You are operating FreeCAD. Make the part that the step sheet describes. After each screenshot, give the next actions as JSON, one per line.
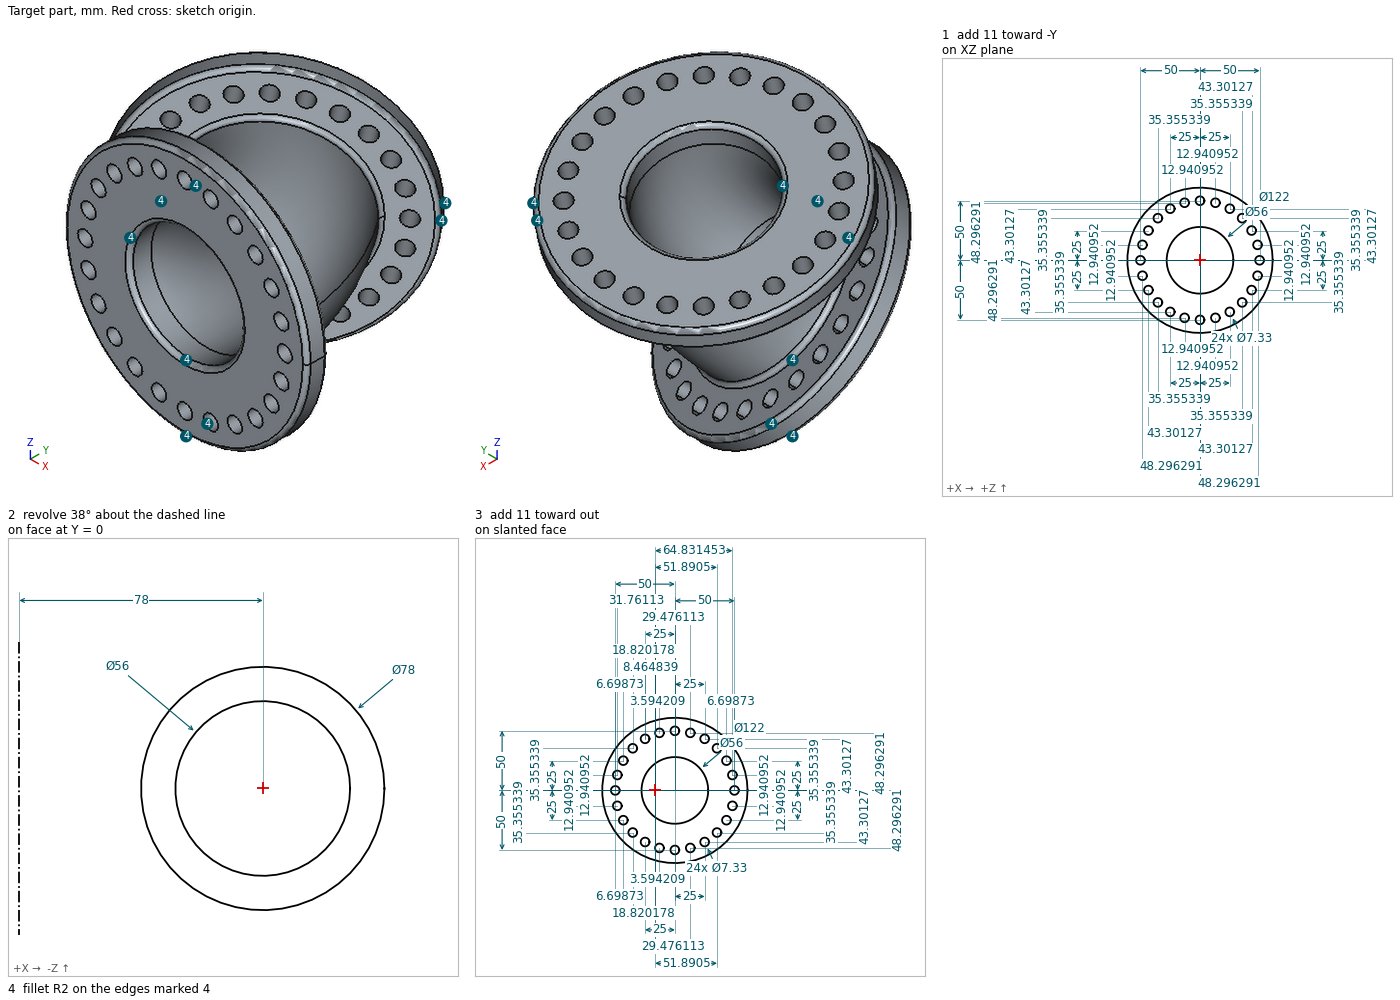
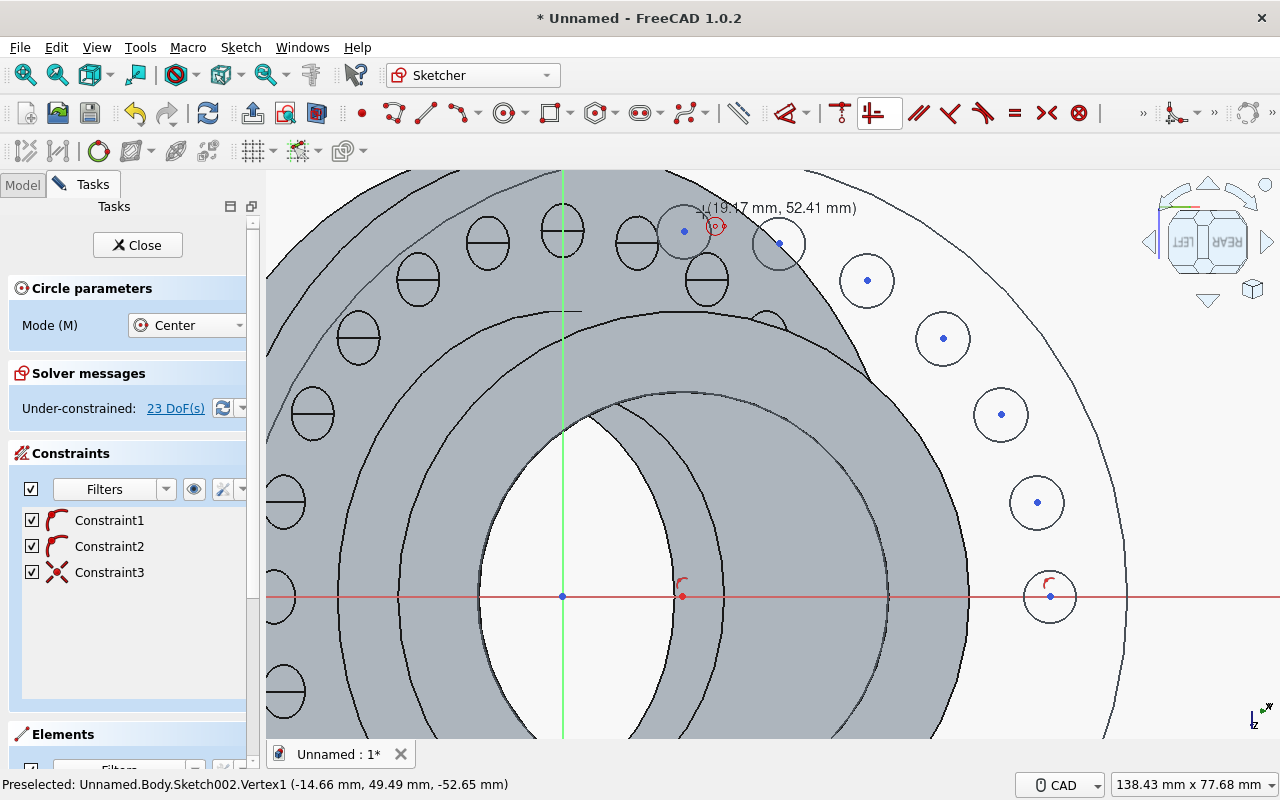
{"action": "left_click", "coordinate": [589, 243]}
{"action": "left_click", "coordinate": [608, 224]}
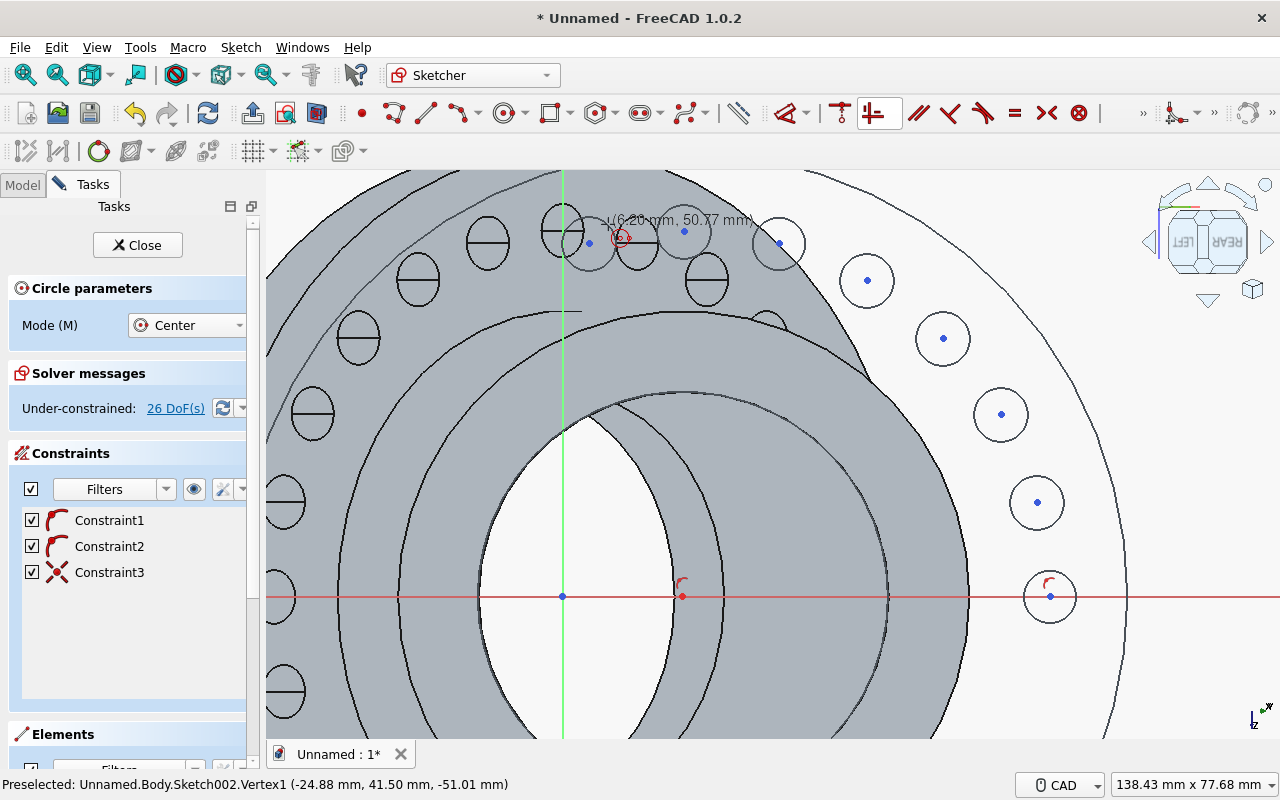
{"action": "left_click", "coordinate": [501, 280]}
{"action": "left_click", "coordinate": [520, 261]}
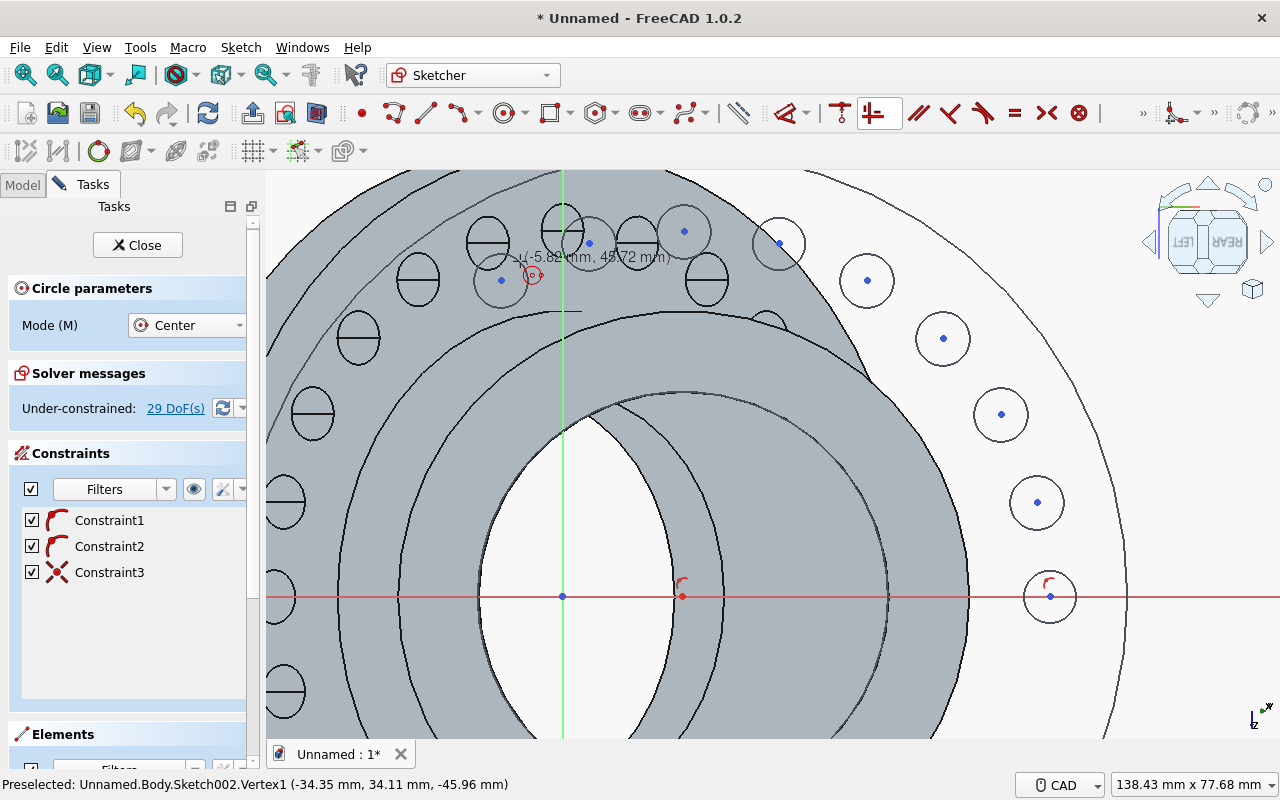
{"action": "left_click", "coordinate": [425, 338]}
{"action": "left_click", "coordinate": [444, 319]}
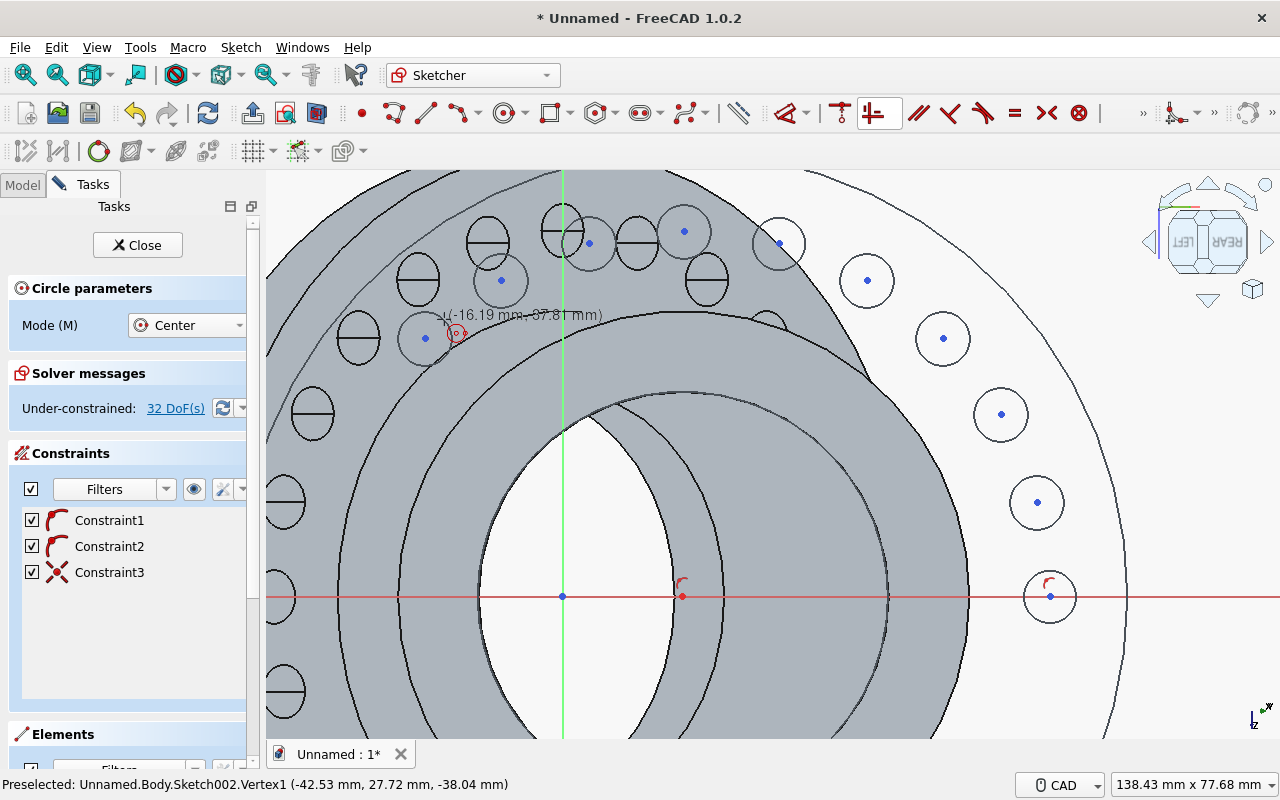
{"action": "left_click", "coordinate": [367, 414]}
{"action": "left_click", "coordinate": [386, 395]}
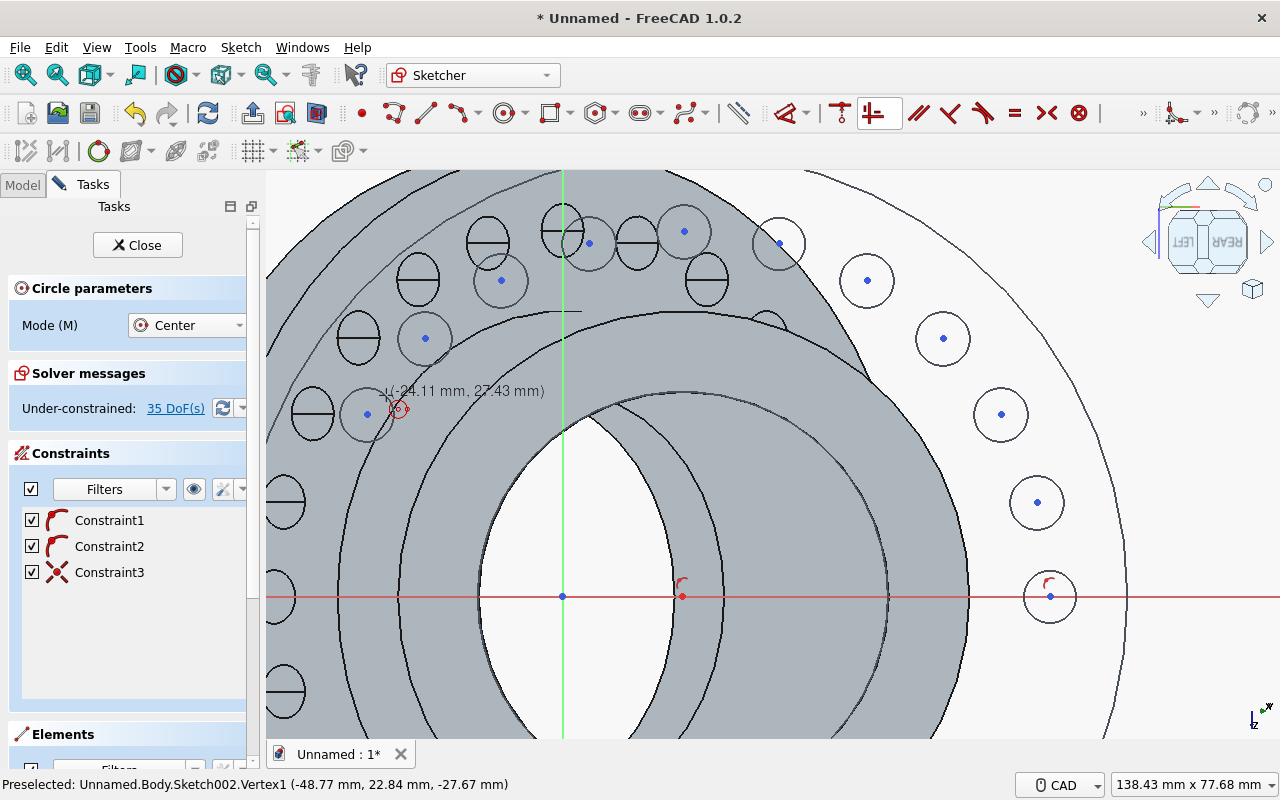
{"action": "left_click", "coordinate": [330, 502]}
{"action": "left_click", "coordinate": [349, 483]}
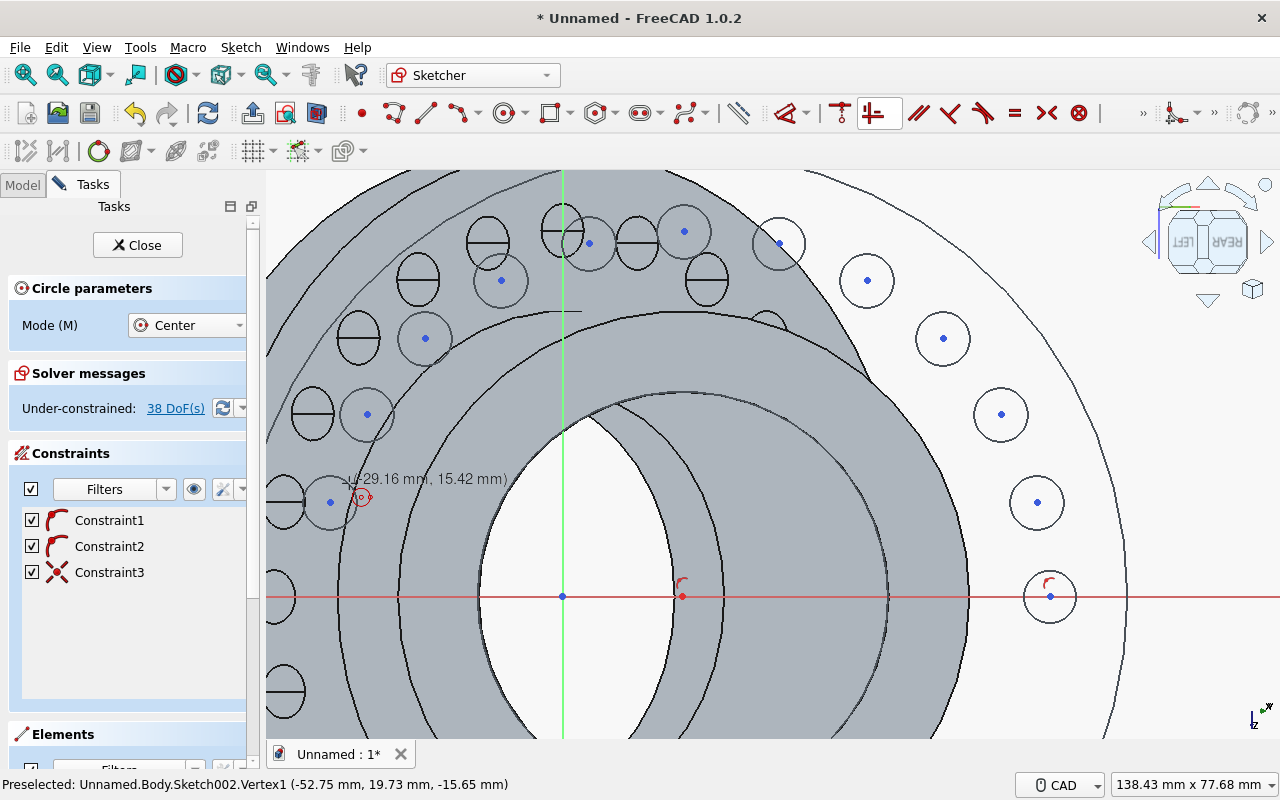
{"action": "left_click", "coordinate": [1037, 692]}
{"action": "left_click", "coordinate": [1056, 673]}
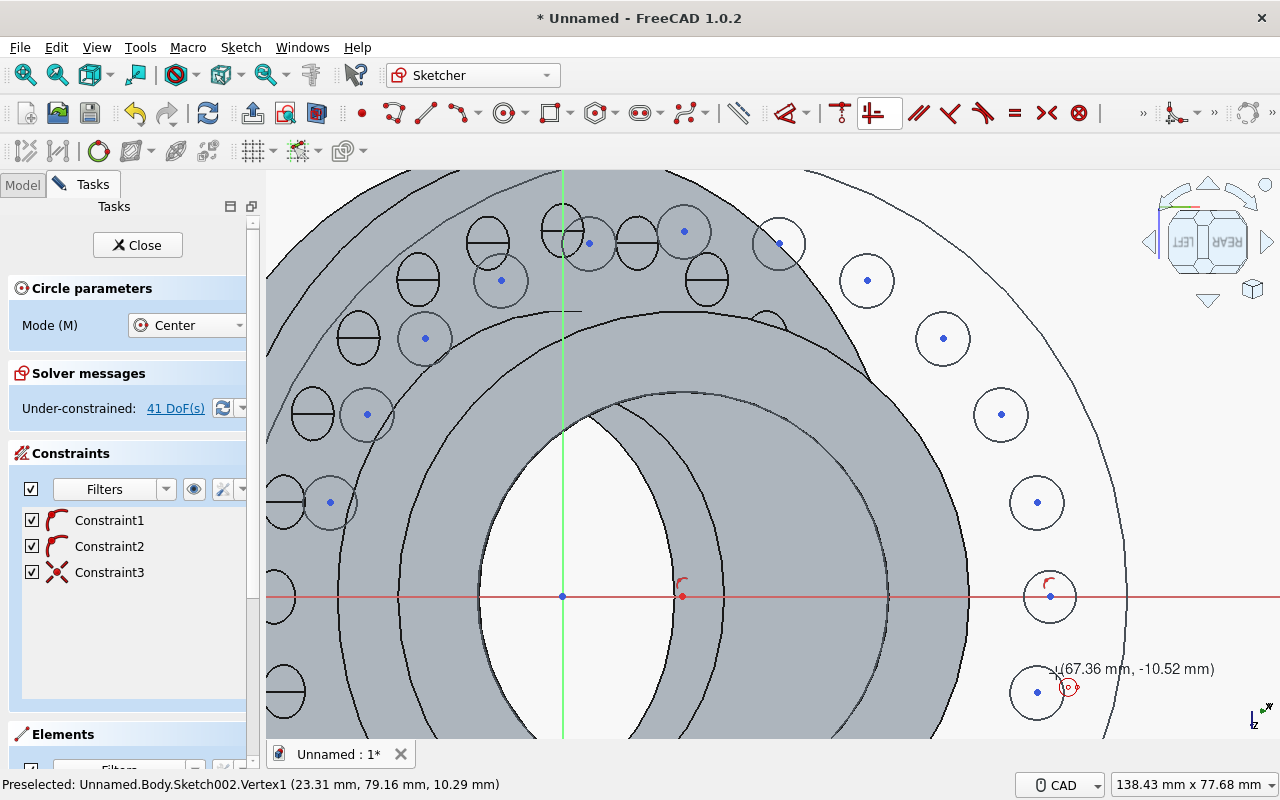
{"action": "scroll", "coordinate": [717, 372], "scroll_direction": "down", "scroll_amount": 5}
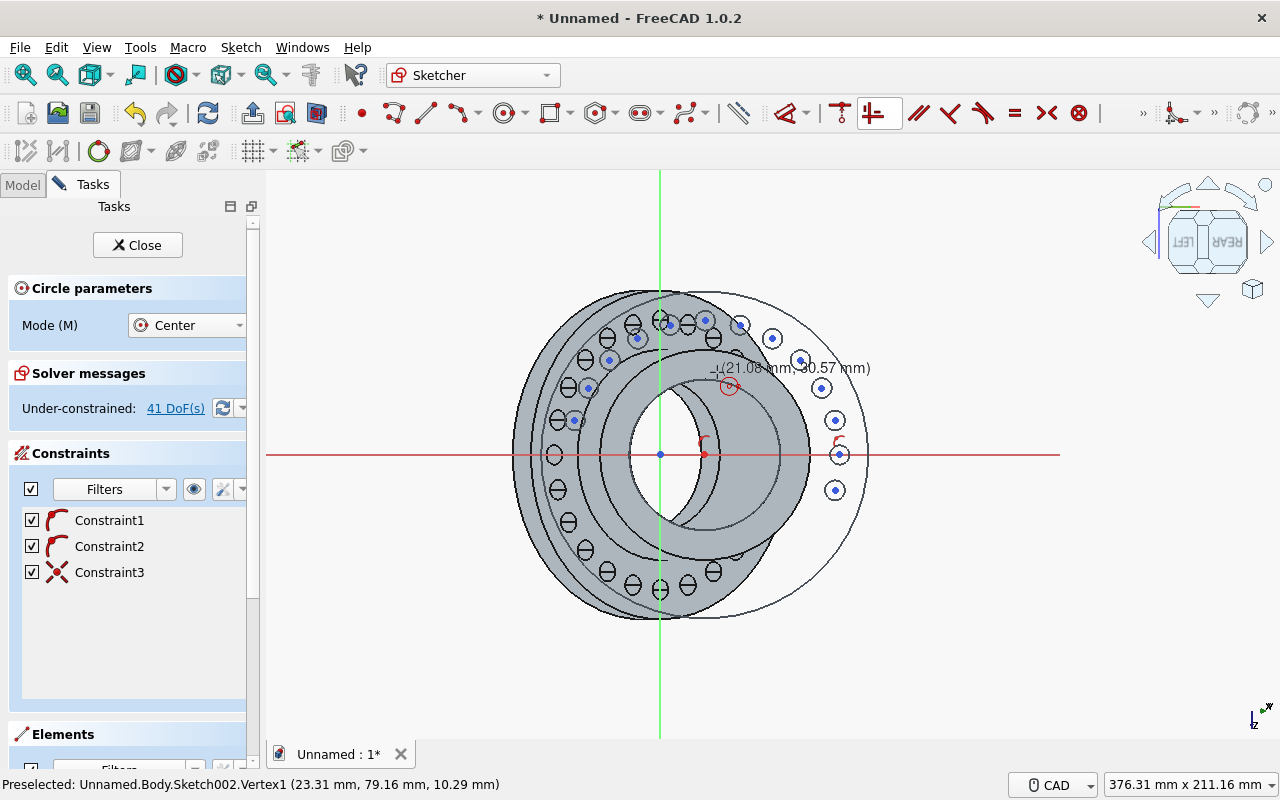
{"action": "scroll", "coordinate": [822, 522], "scroll_direction": "up", "scroll_amount": 5}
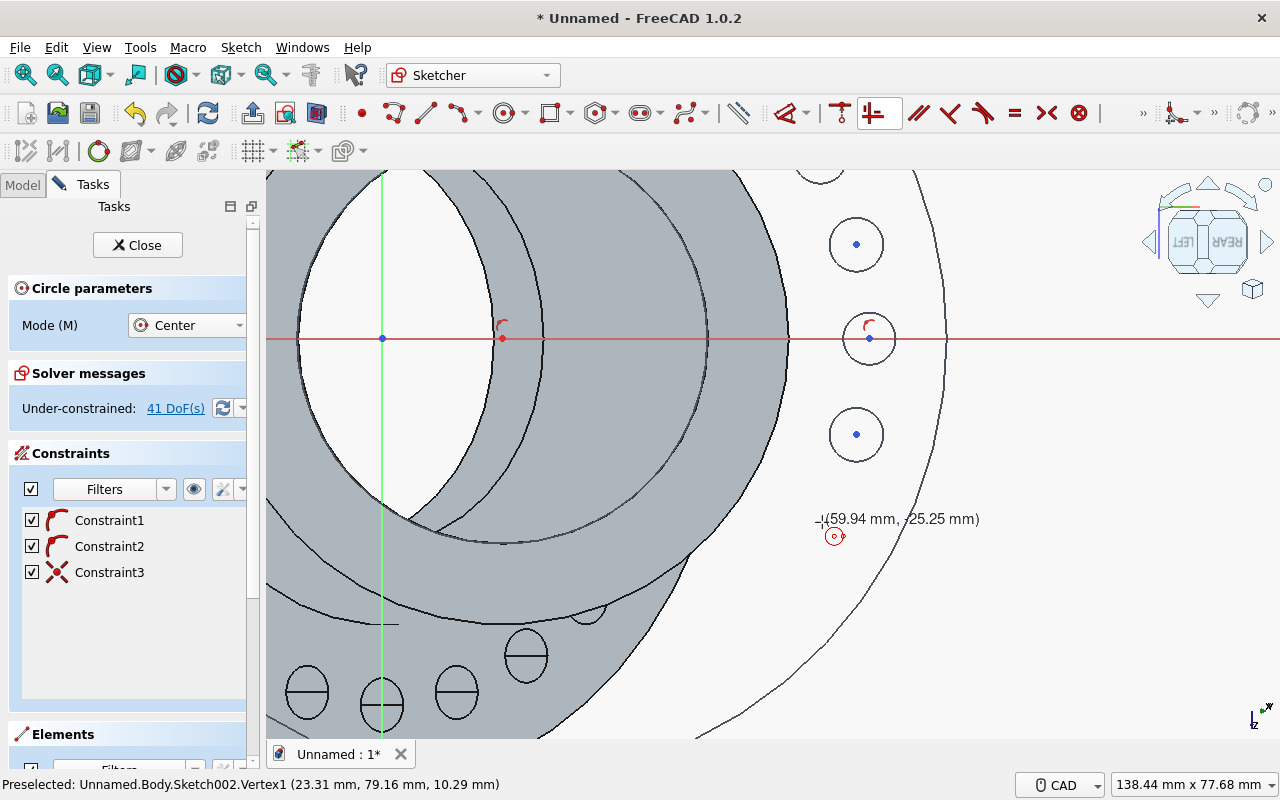
{"action": "left_click", "coordinate": [820, 522]}
{"action": "left_click", "coordinate": [839, 503]}